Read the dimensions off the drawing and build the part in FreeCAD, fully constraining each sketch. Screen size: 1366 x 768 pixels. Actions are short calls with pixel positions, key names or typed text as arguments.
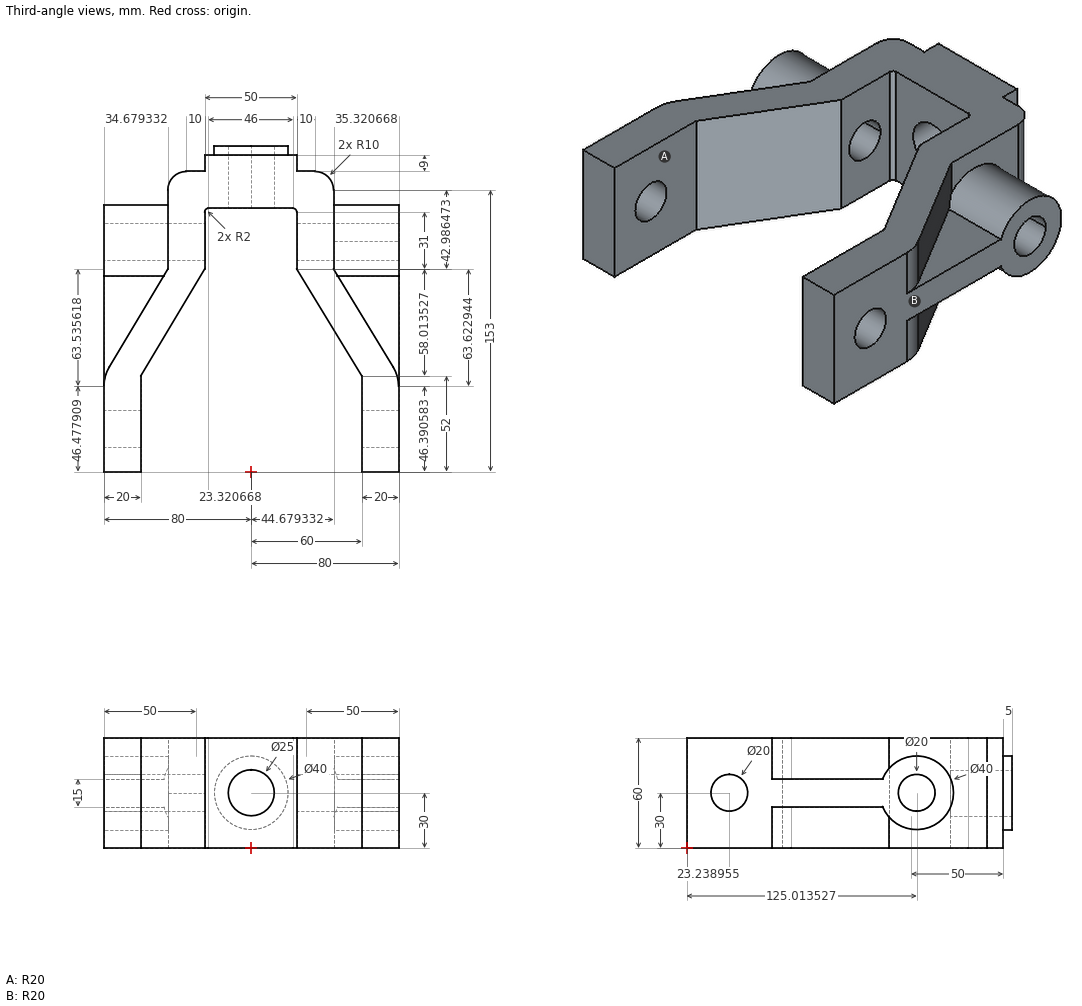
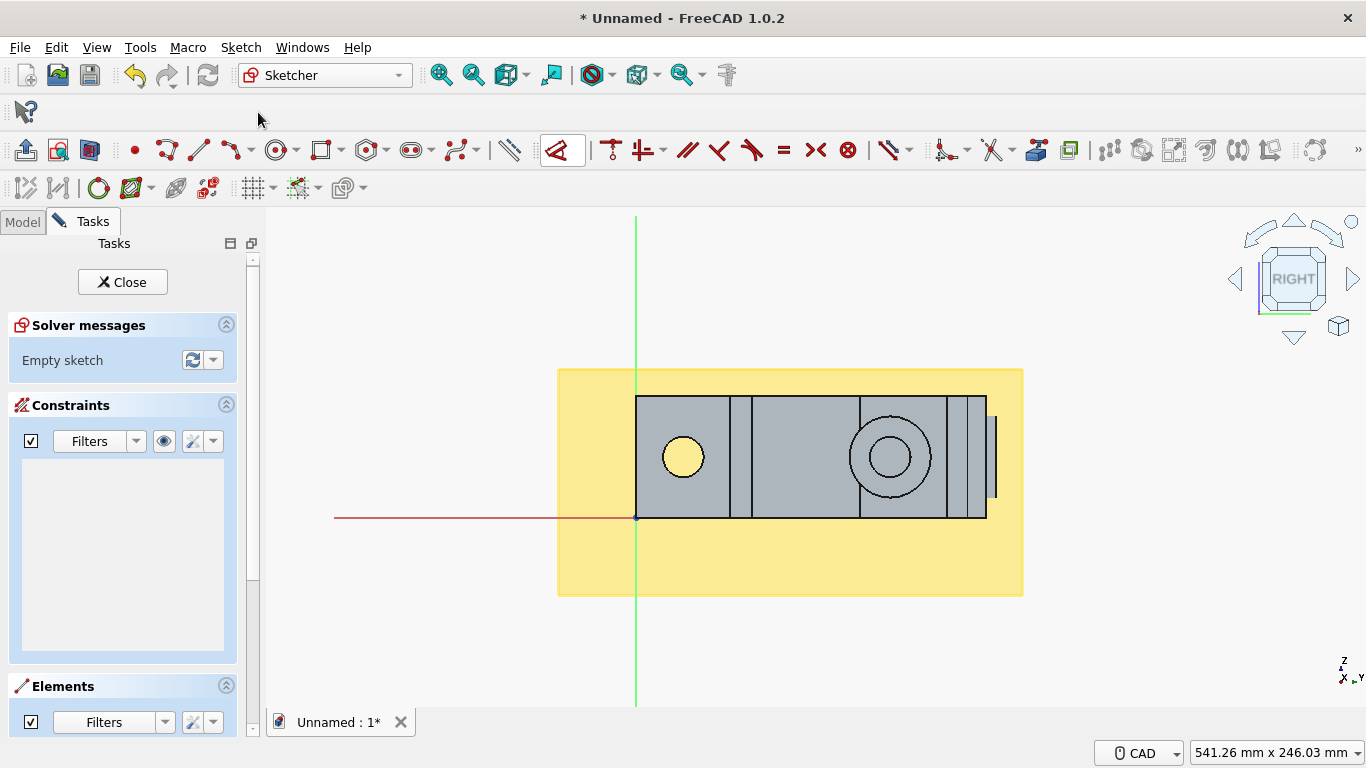
key(q)
key(s)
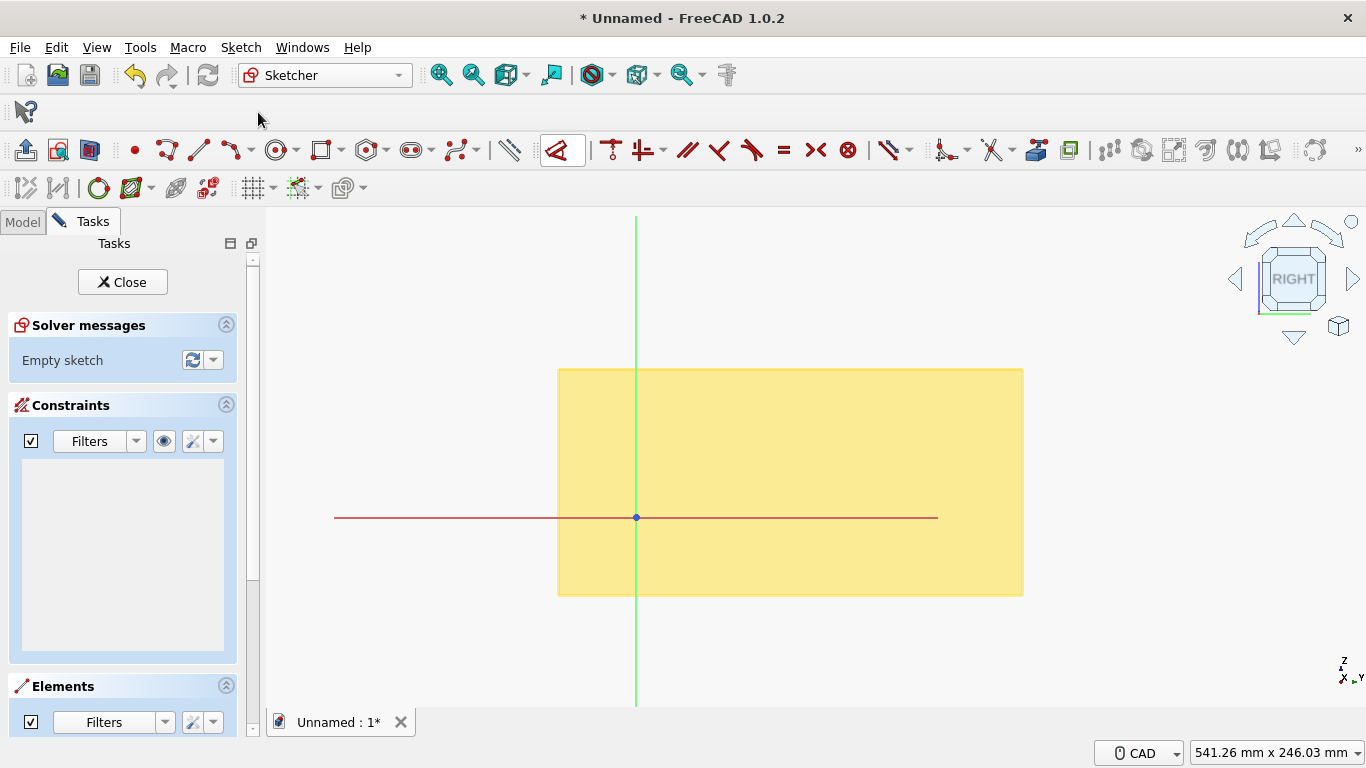
scroll(913, 457, up, 10)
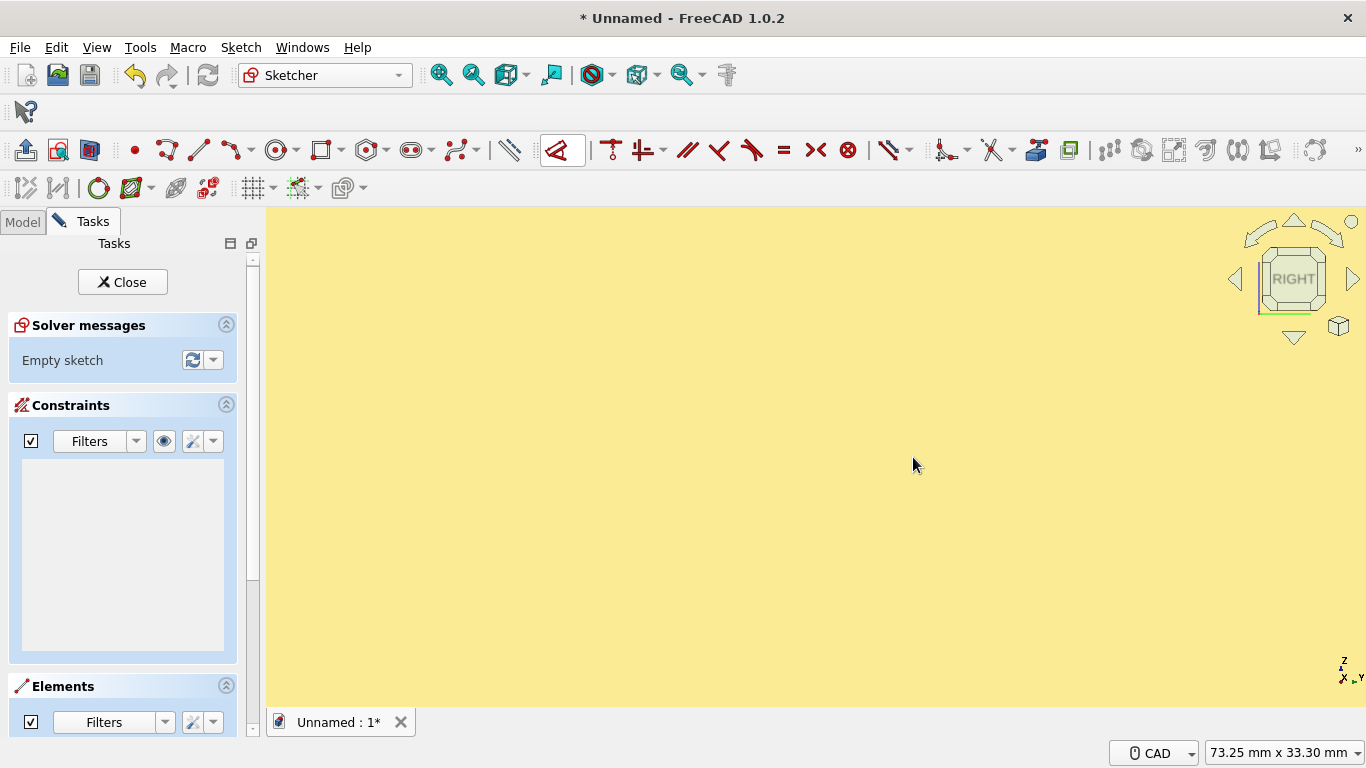
key(g)
key(c)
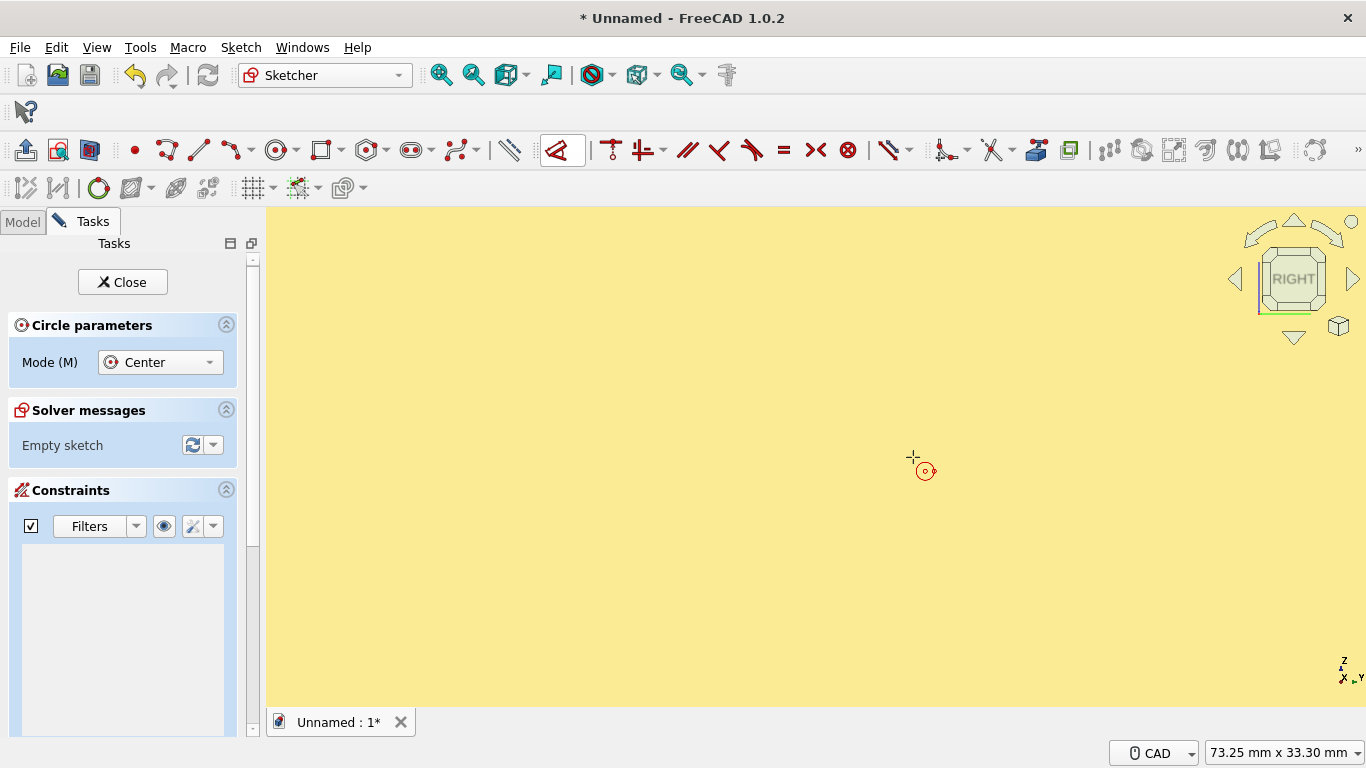
click(741, 454)
click(847, 348)
key(Escape)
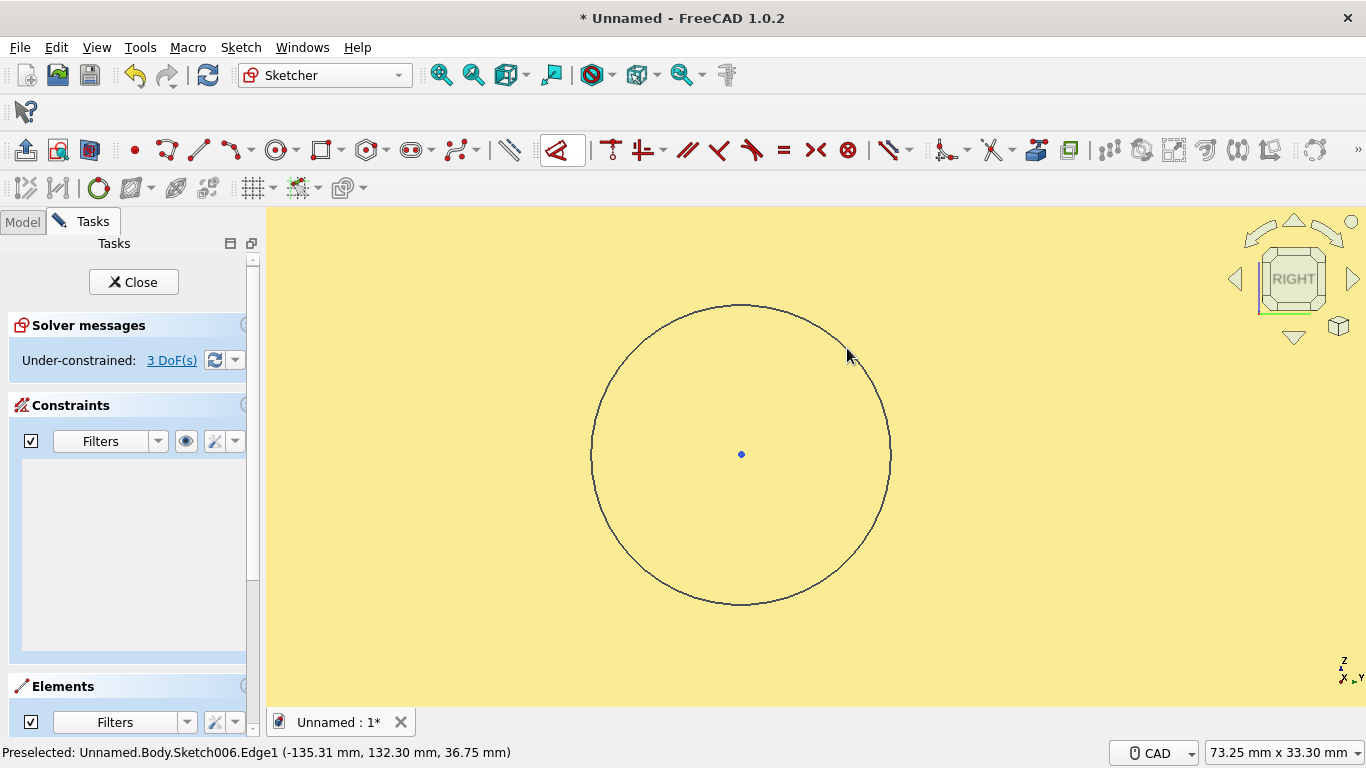
click(847, 349)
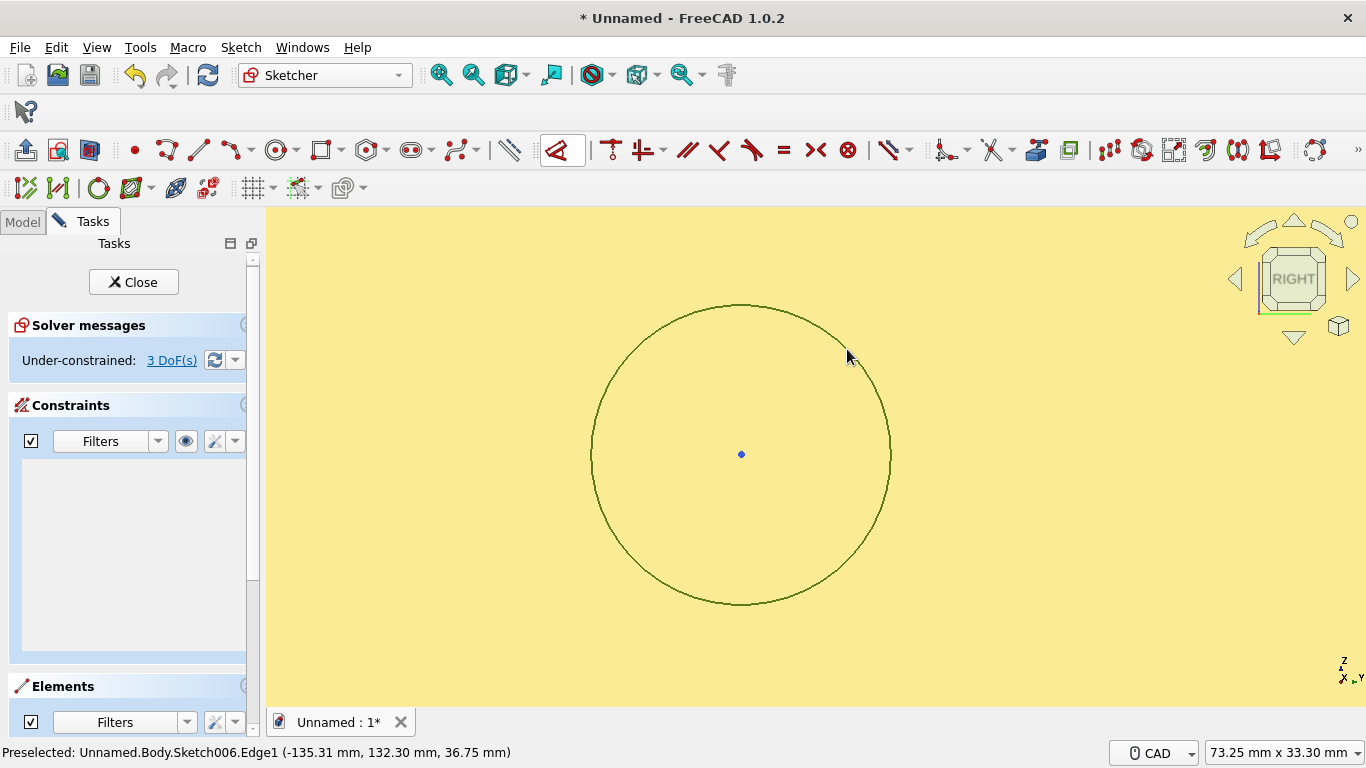
key(k)
key(o)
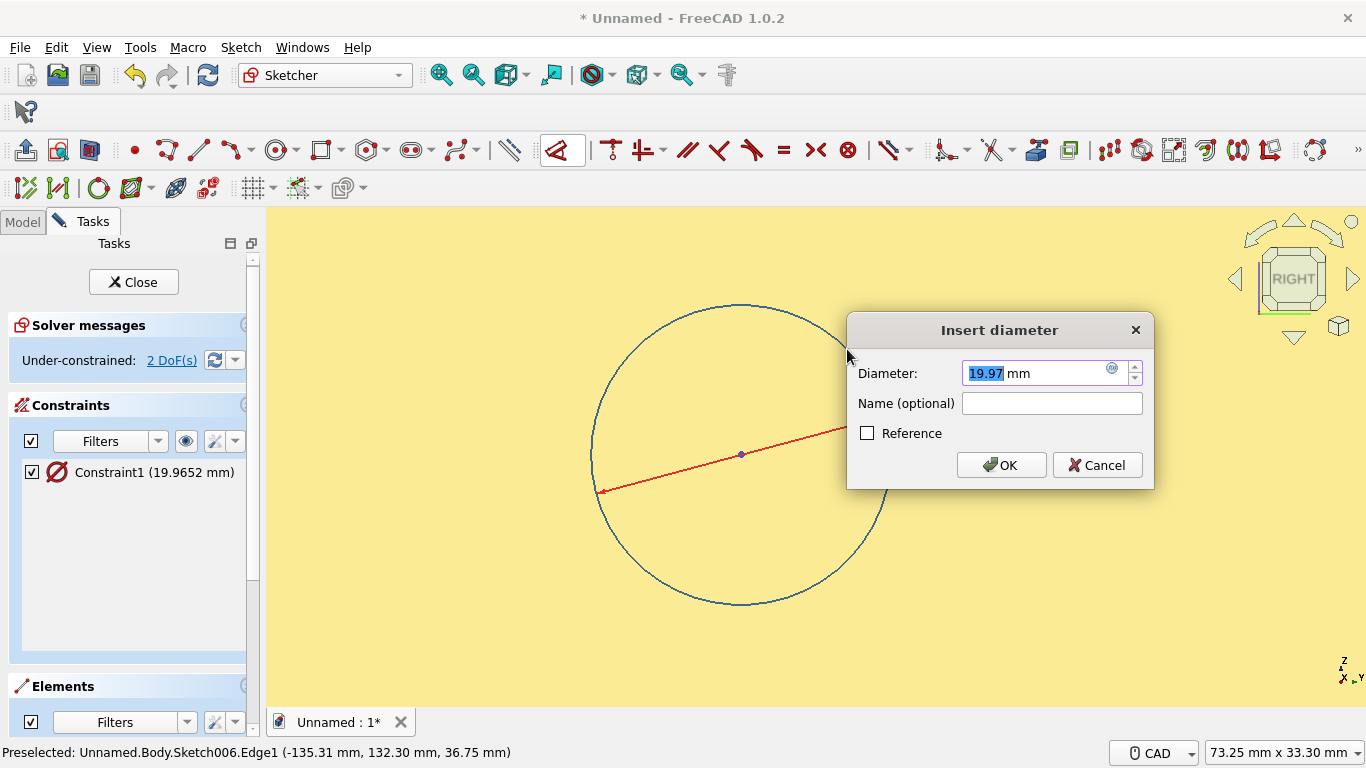
text(20)
key(Return)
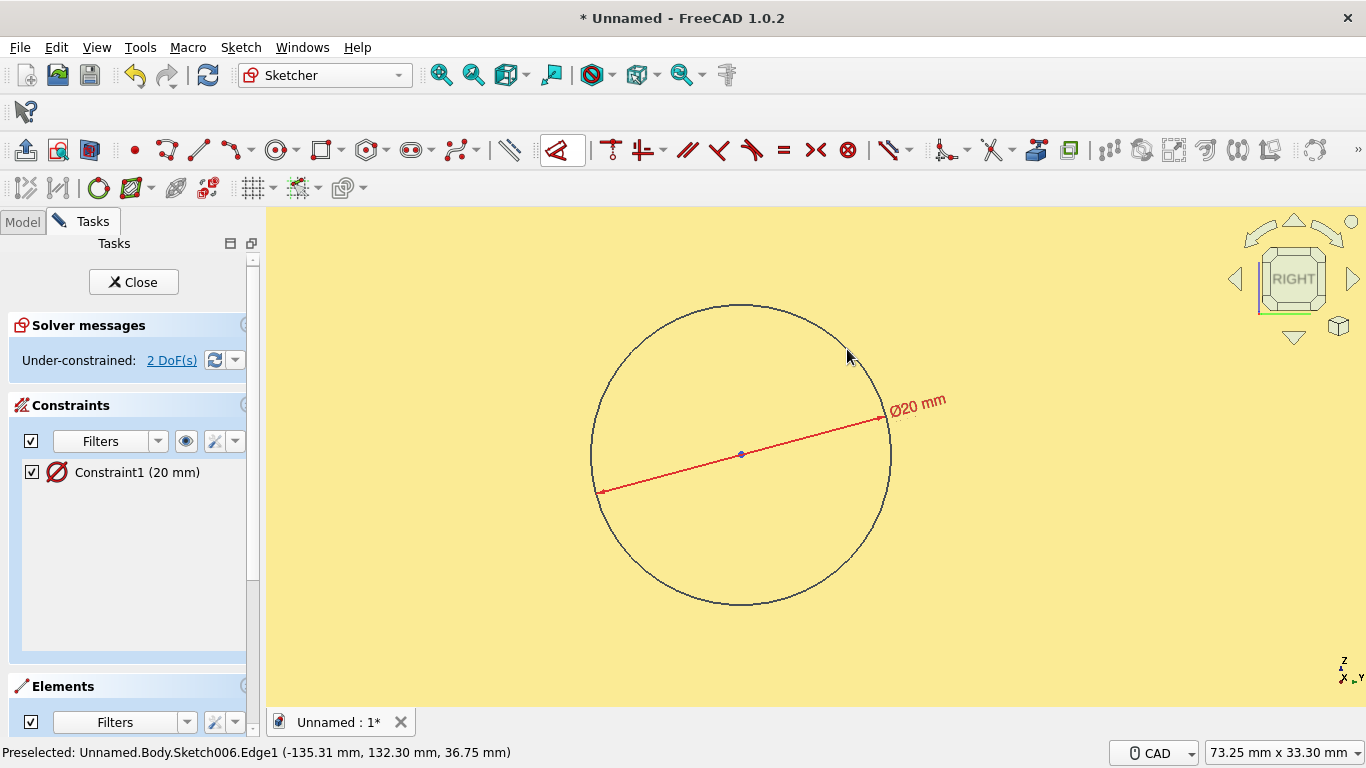
click(741, 455)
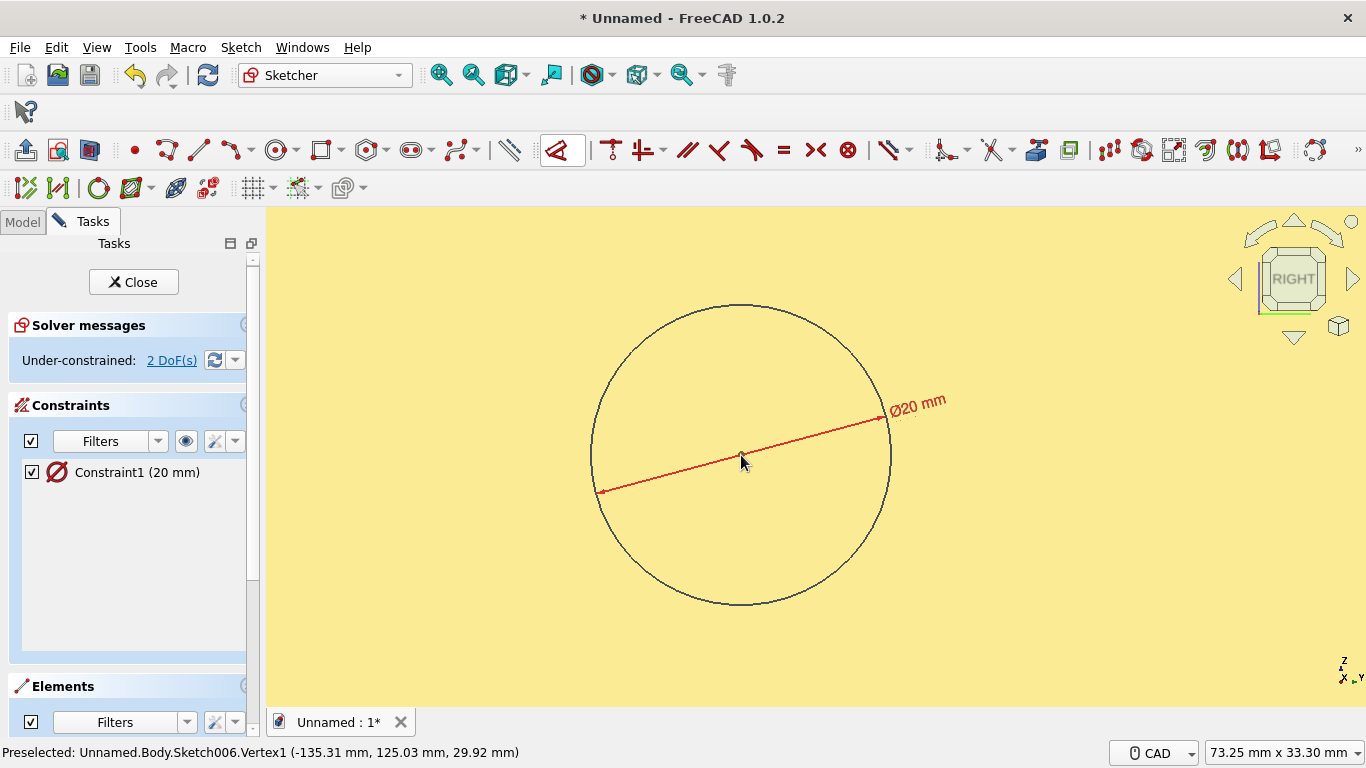
key(i)